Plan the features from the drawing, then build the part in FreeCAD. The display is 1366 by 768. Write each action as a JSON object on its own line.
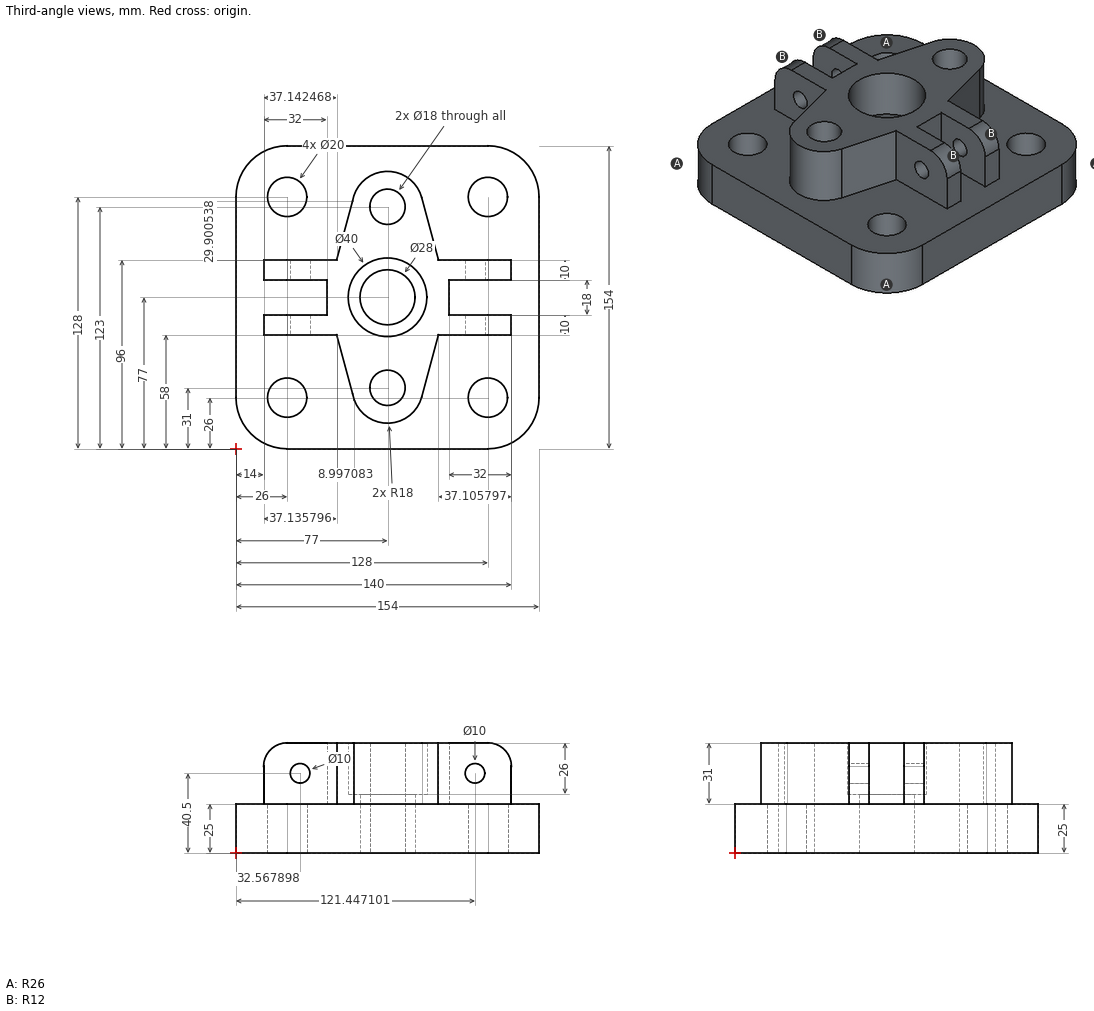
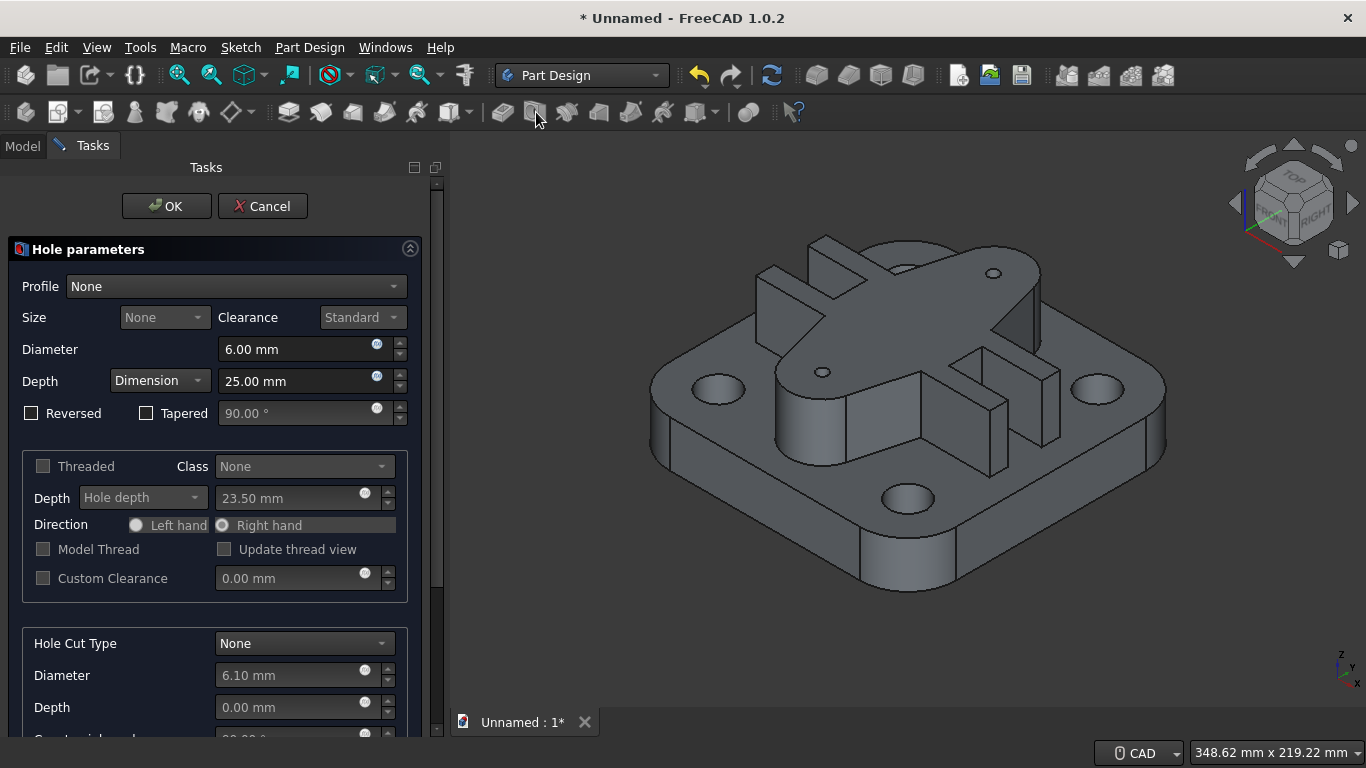
{"action": "triple_click", "coordinate": [305, 349]}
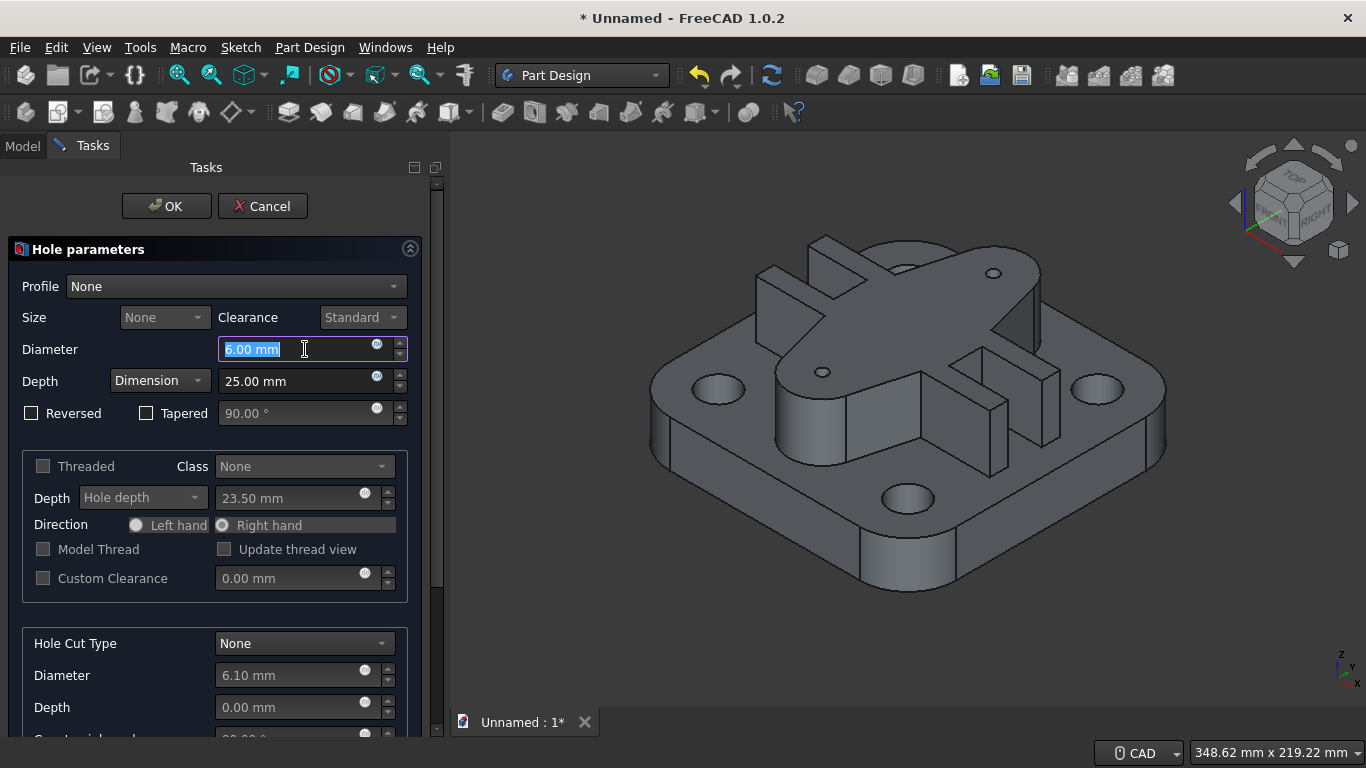
{"action": "type", "text": "18"}
{"action": "key", "text": "Tab"}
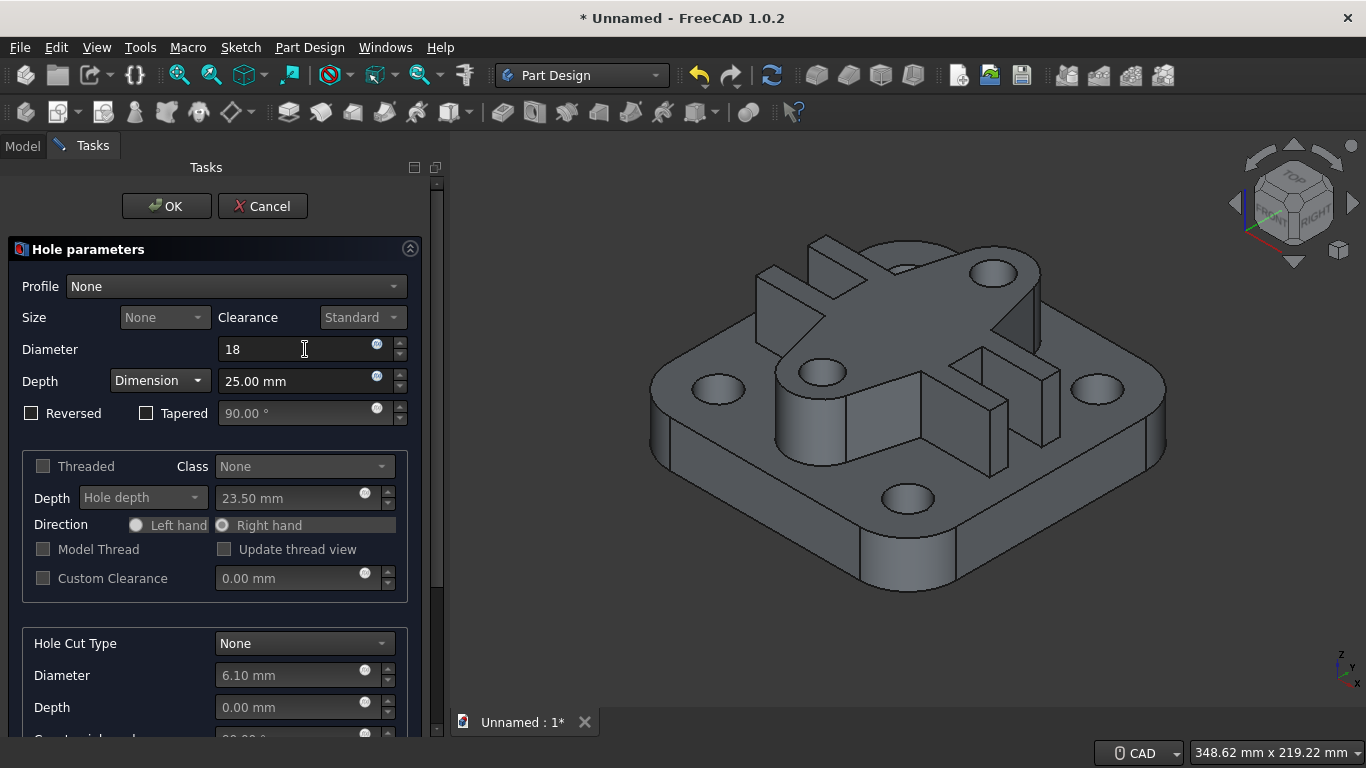
{"action": "left_click", "coordinate": [161, 380]}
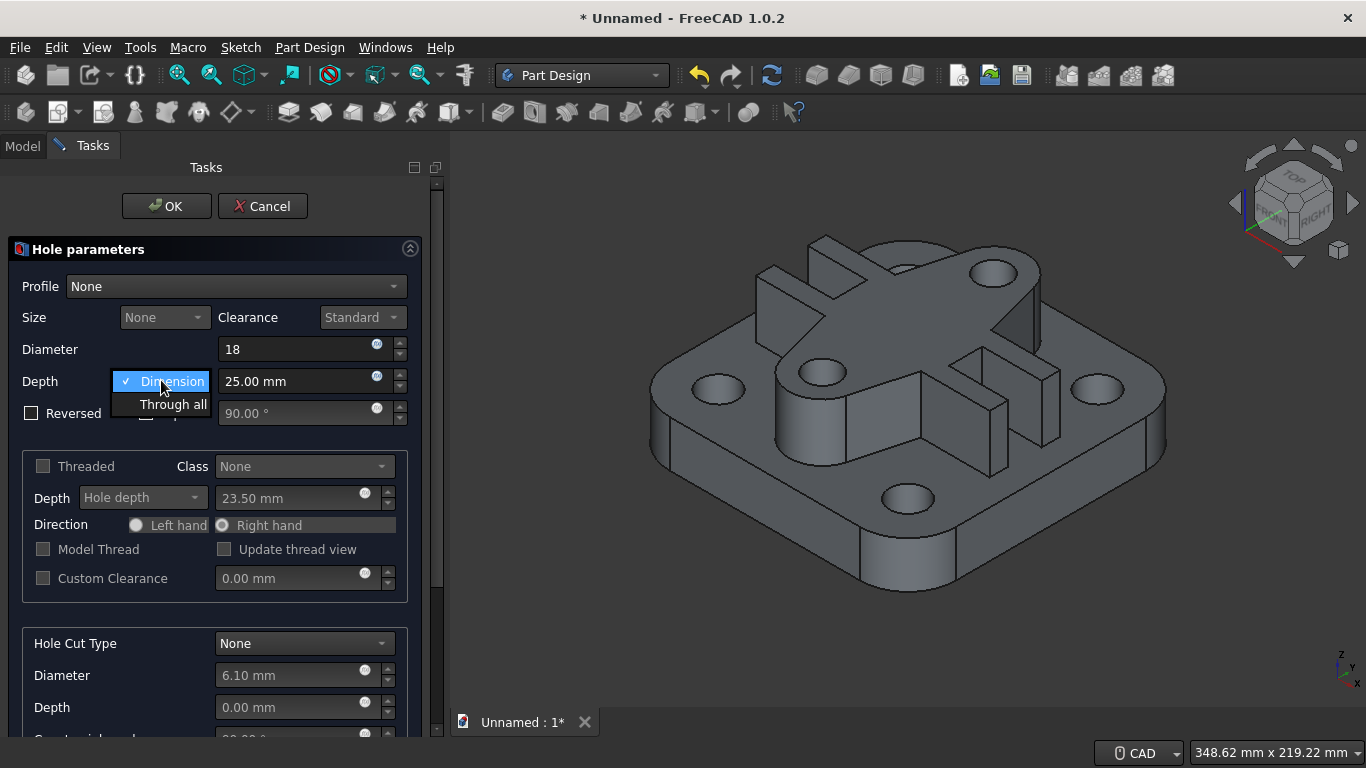
{"action": "left_click", "coordinate": [160, 404]}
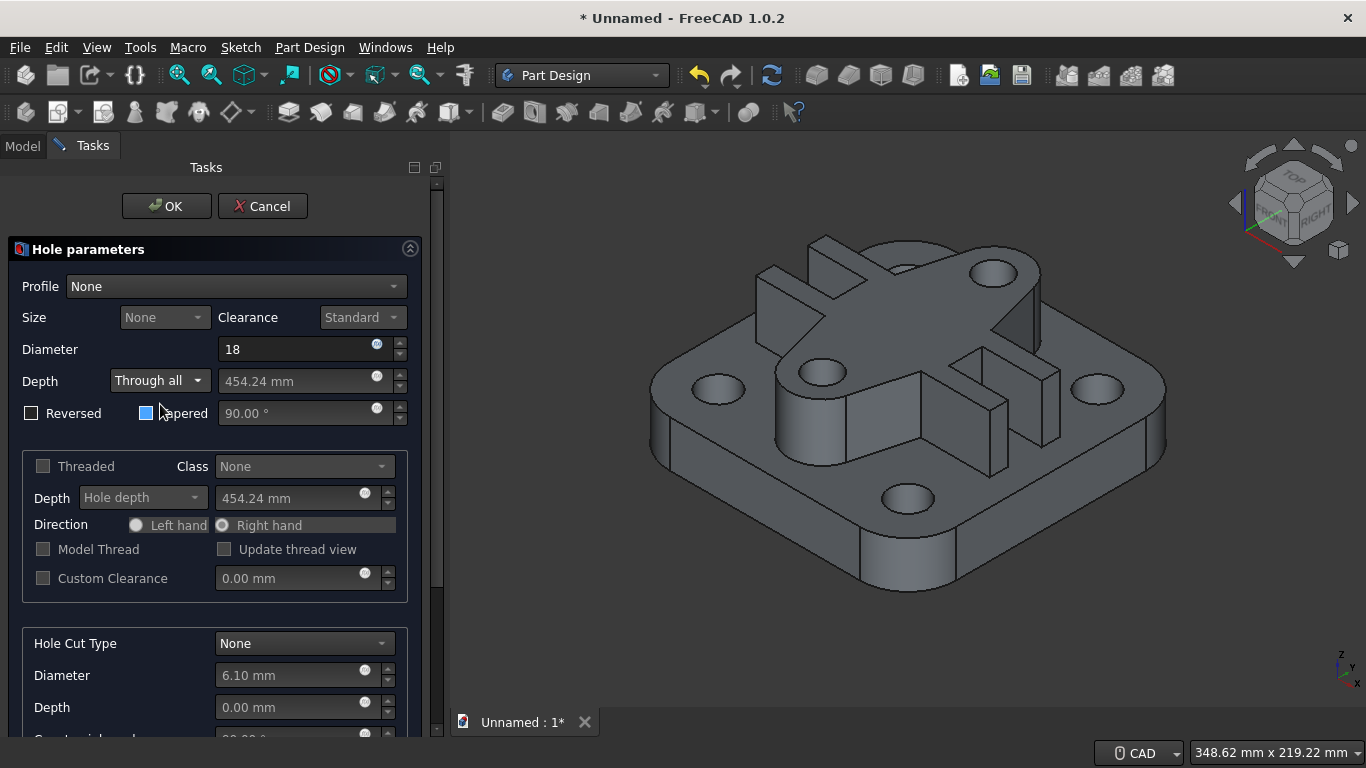
{"action": "left_click", "coordinate": [167, 206]}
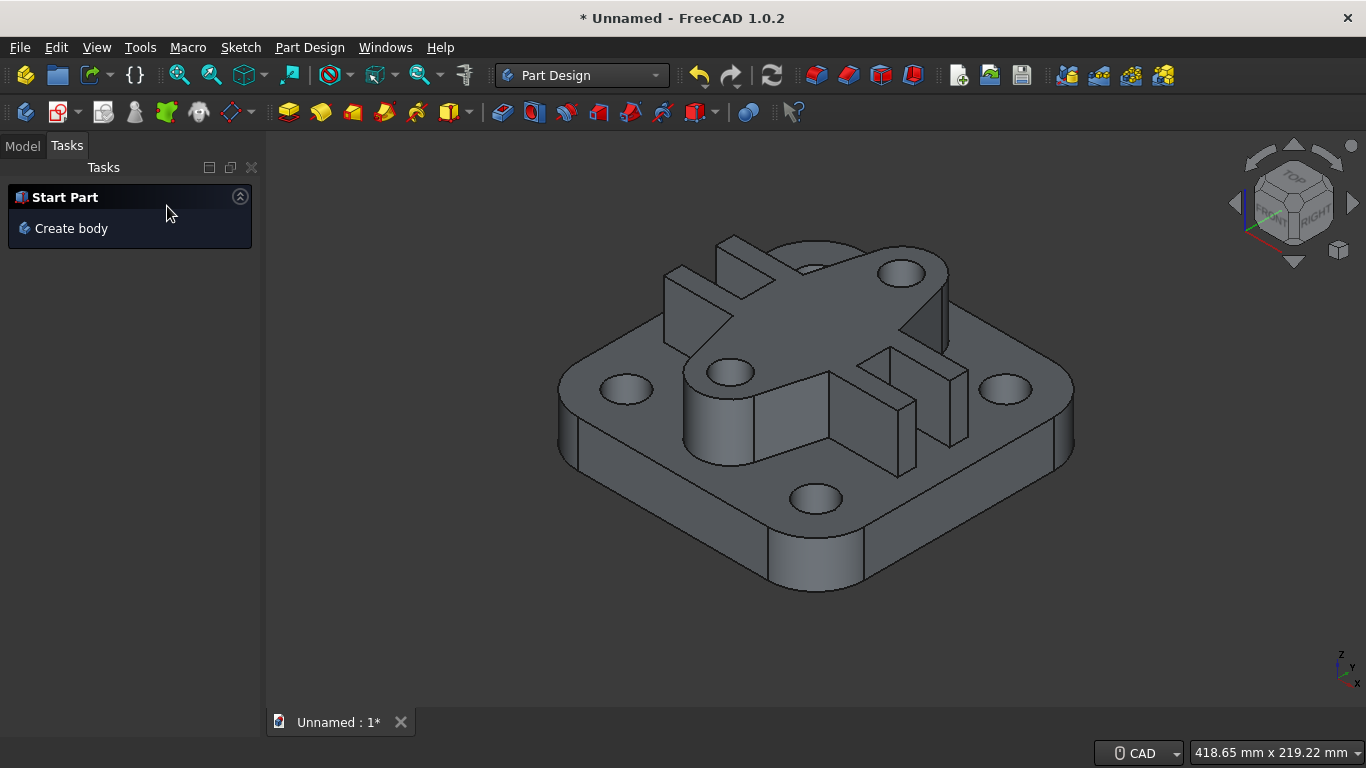
{"action": "left_click", "coordinate": [816, 322]}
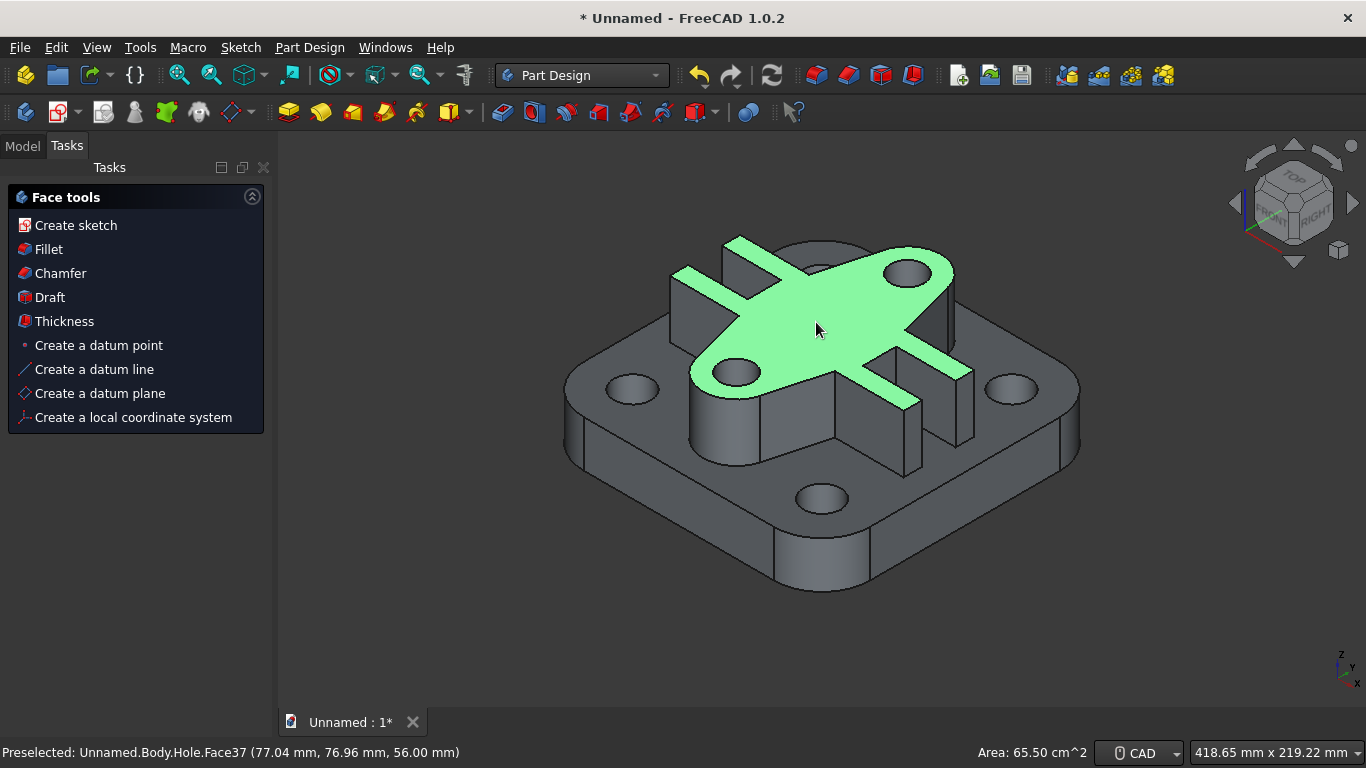
{"action": "left_click", "coordinate": [58, 112]}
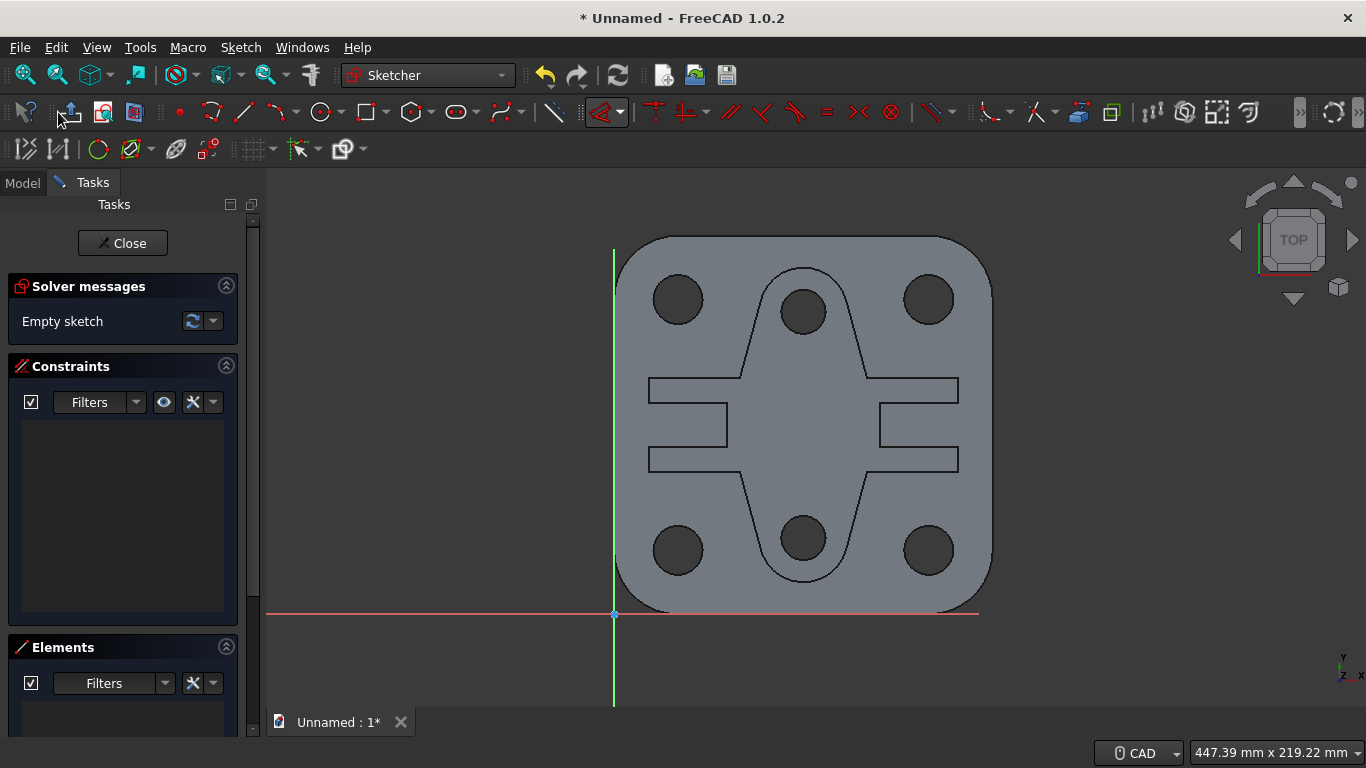
{"action": "scroll", "coordinate": [818, 422], "scroll_direction": "up", "scroll_amount": 8}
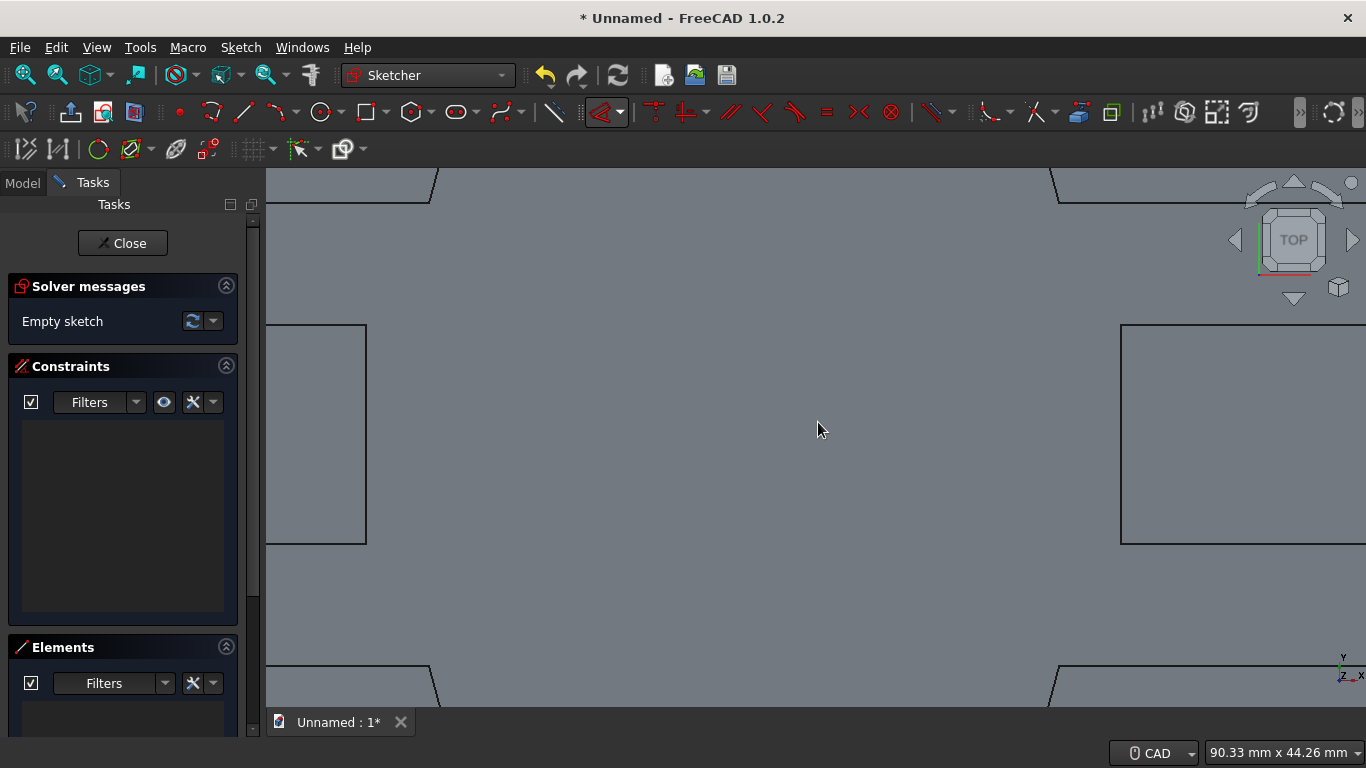
{"action": "left_click", "coordinate": [322, 112]}